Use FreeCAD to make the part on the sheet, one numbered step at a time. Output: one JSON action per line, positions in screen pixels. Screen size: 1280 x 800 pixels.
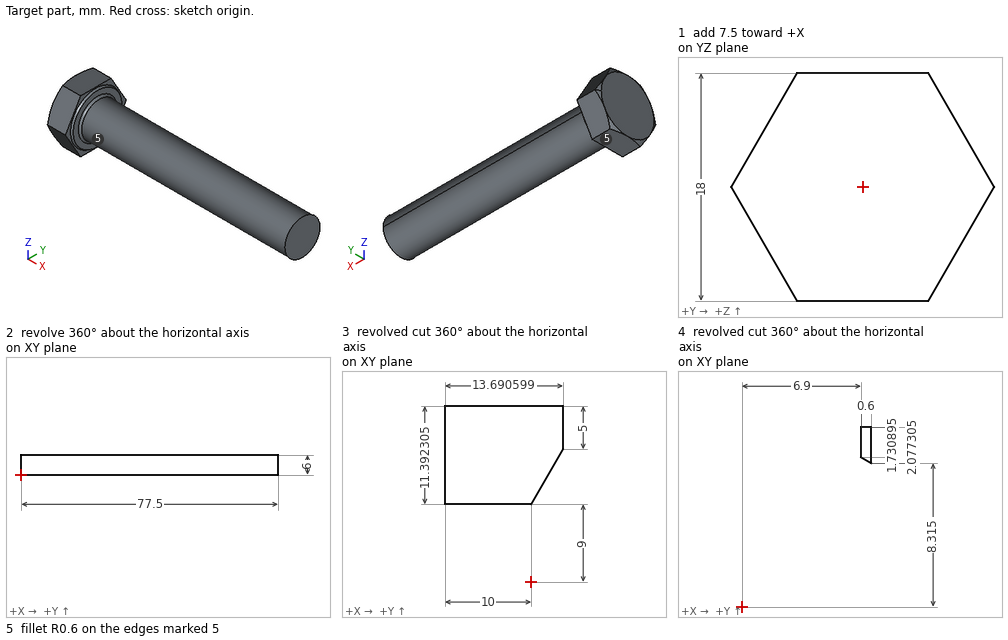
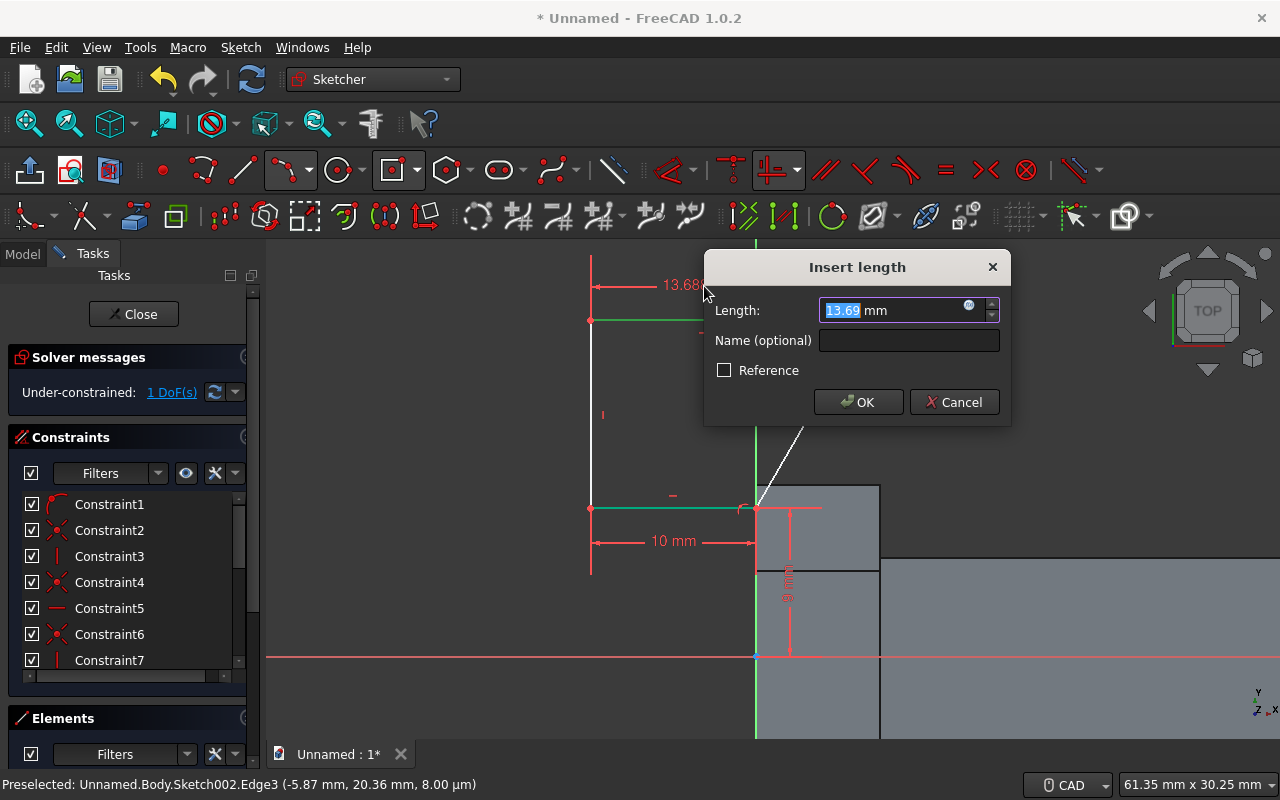
{"action": "type", "text": "13.690599"}
{"action": "key", "text": "Return"}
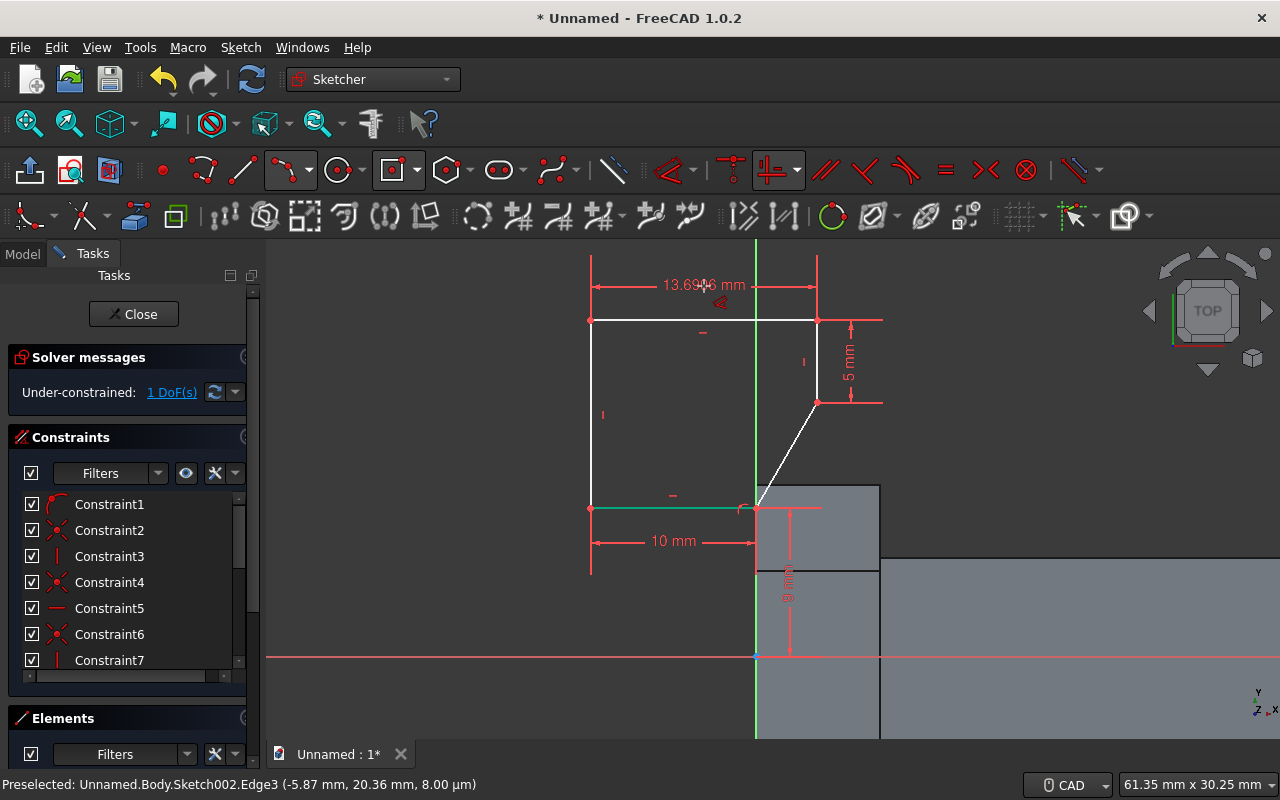
{"action": "left_click", "coordinate": [591, 377]}
{"action": "left_click", "coordinate": [557, 414]}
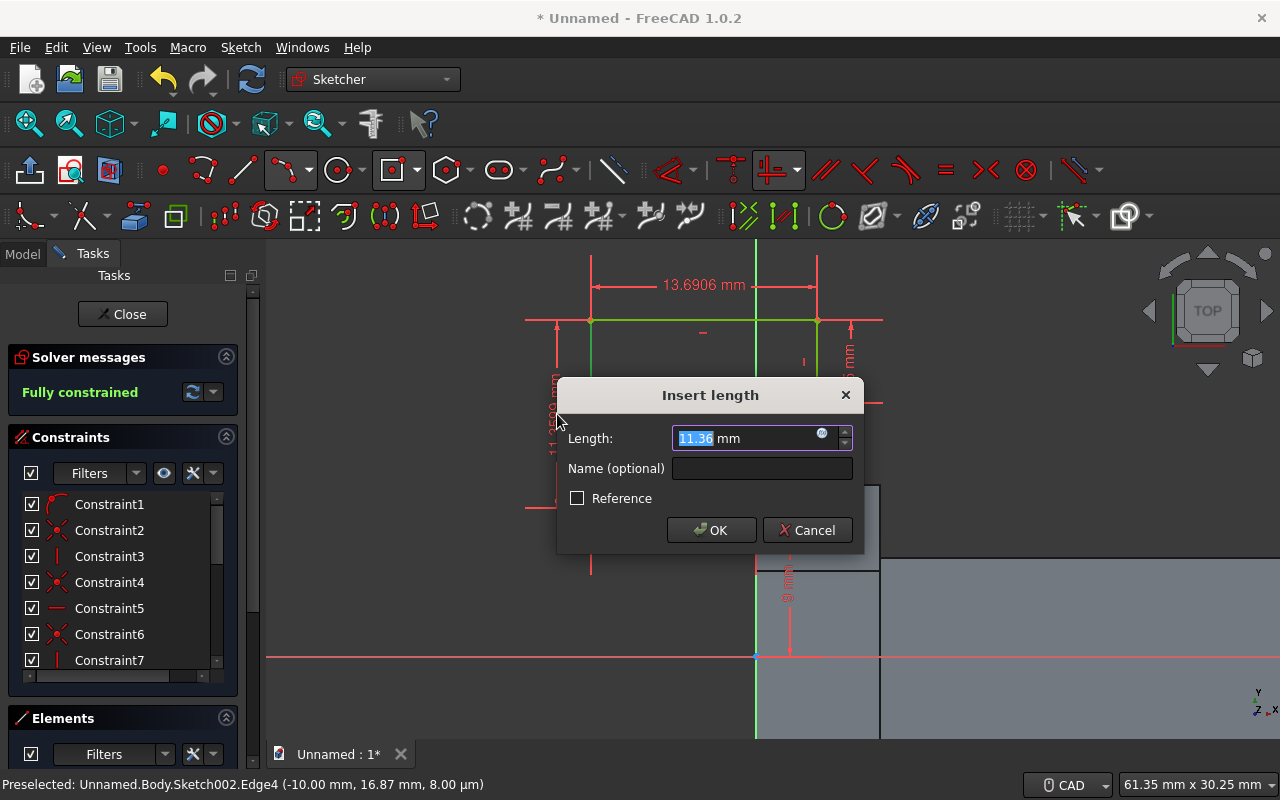
{"action": "type", "text": "11.392305"}
{"action": "key", "text": "Return"}
{"action": "key", "text": "Escape"}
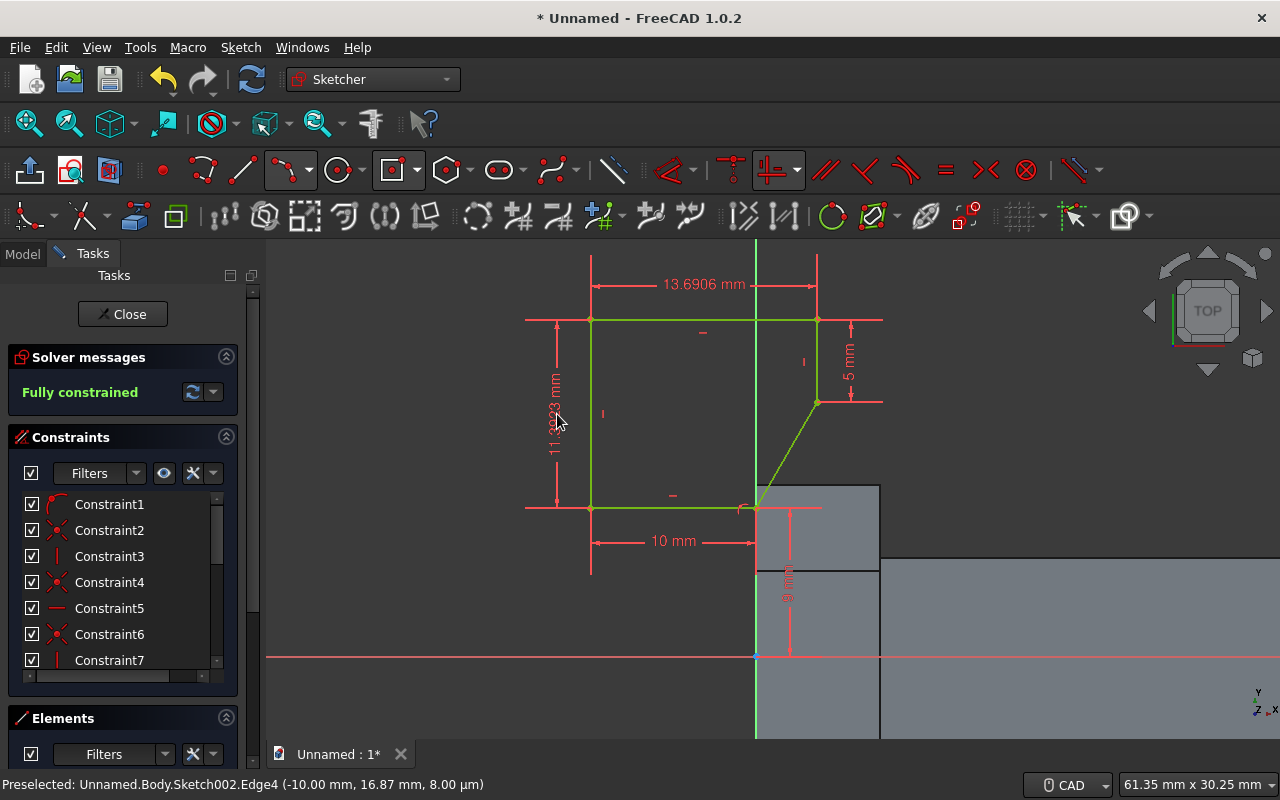
{"action": "left_click", "coordinate": [123, 314]}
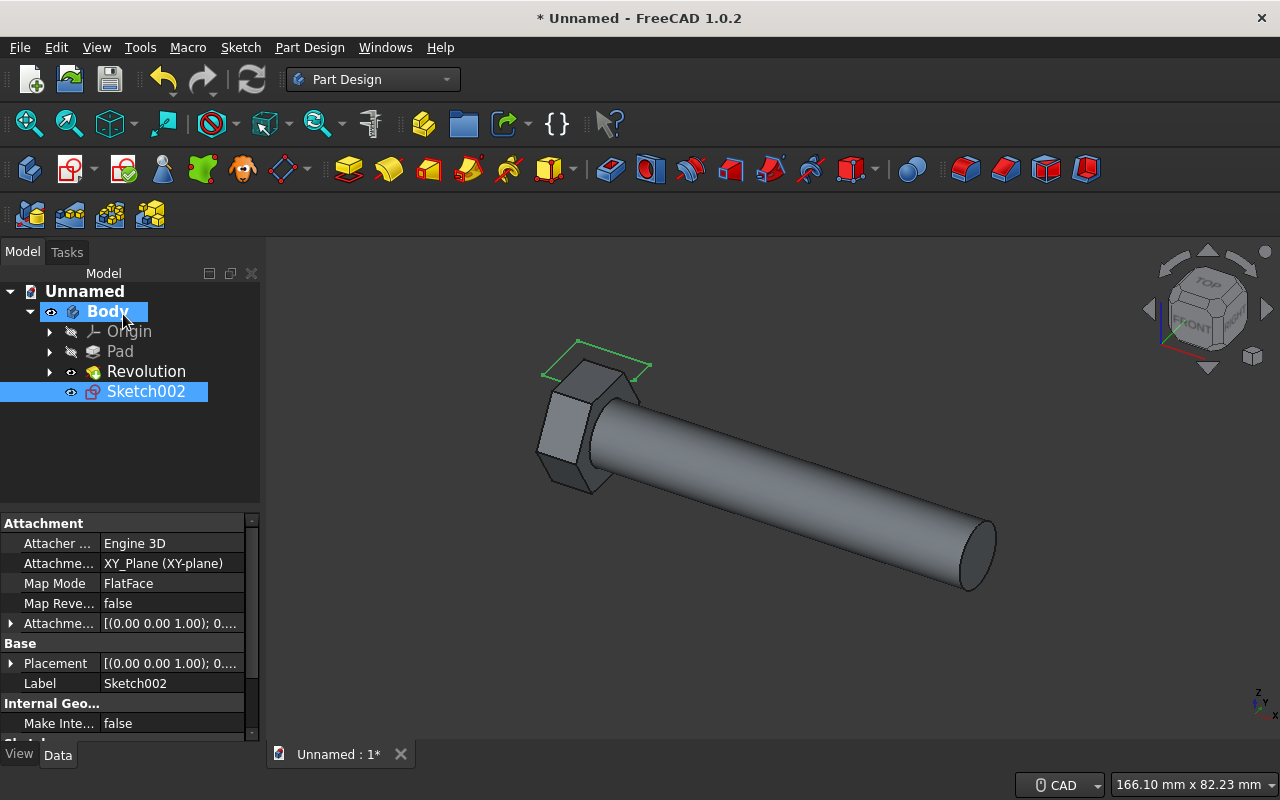
{"action": "left_click", "coordinate": [692, 170]}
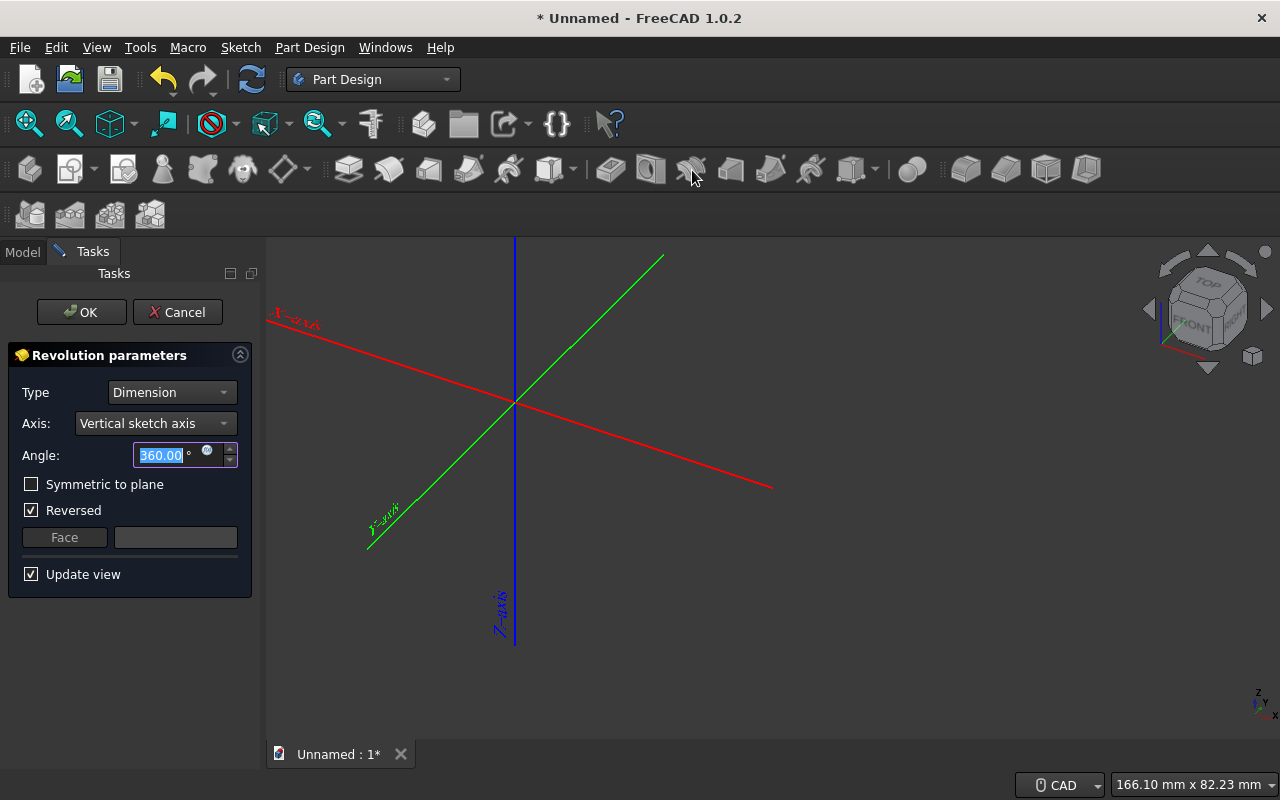
{"action": "left_click", "coordinate": [156, 424]}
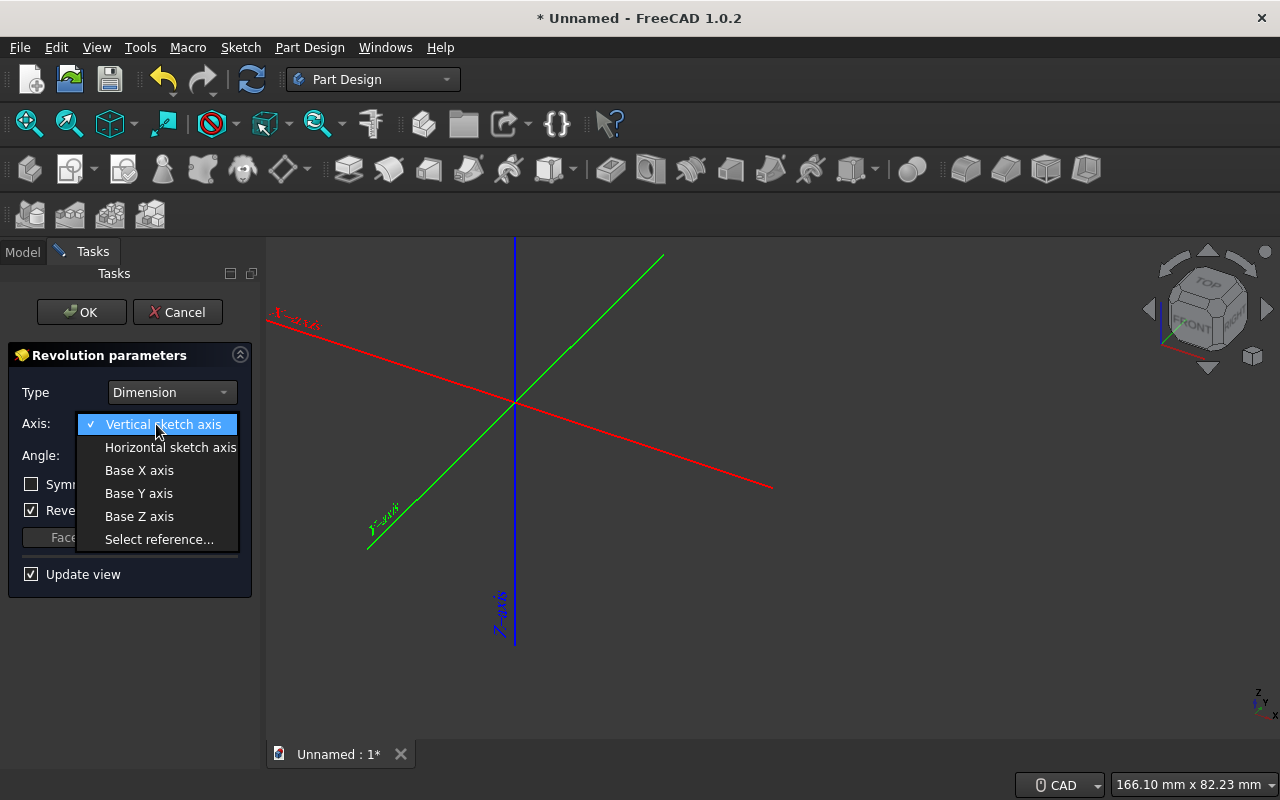
{"action": "left_click", "coordinate": [156, 448]}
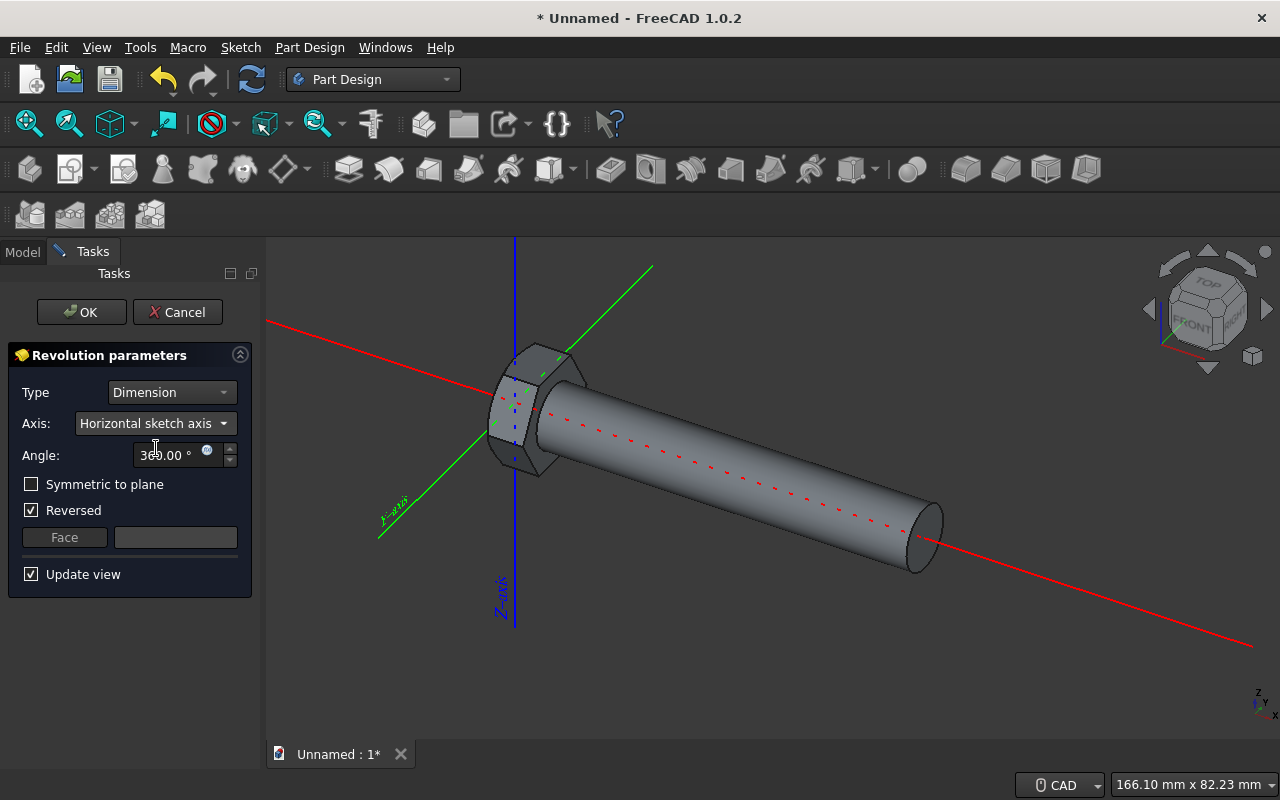
{"action": "left_click", "coordinate": [82, 312]}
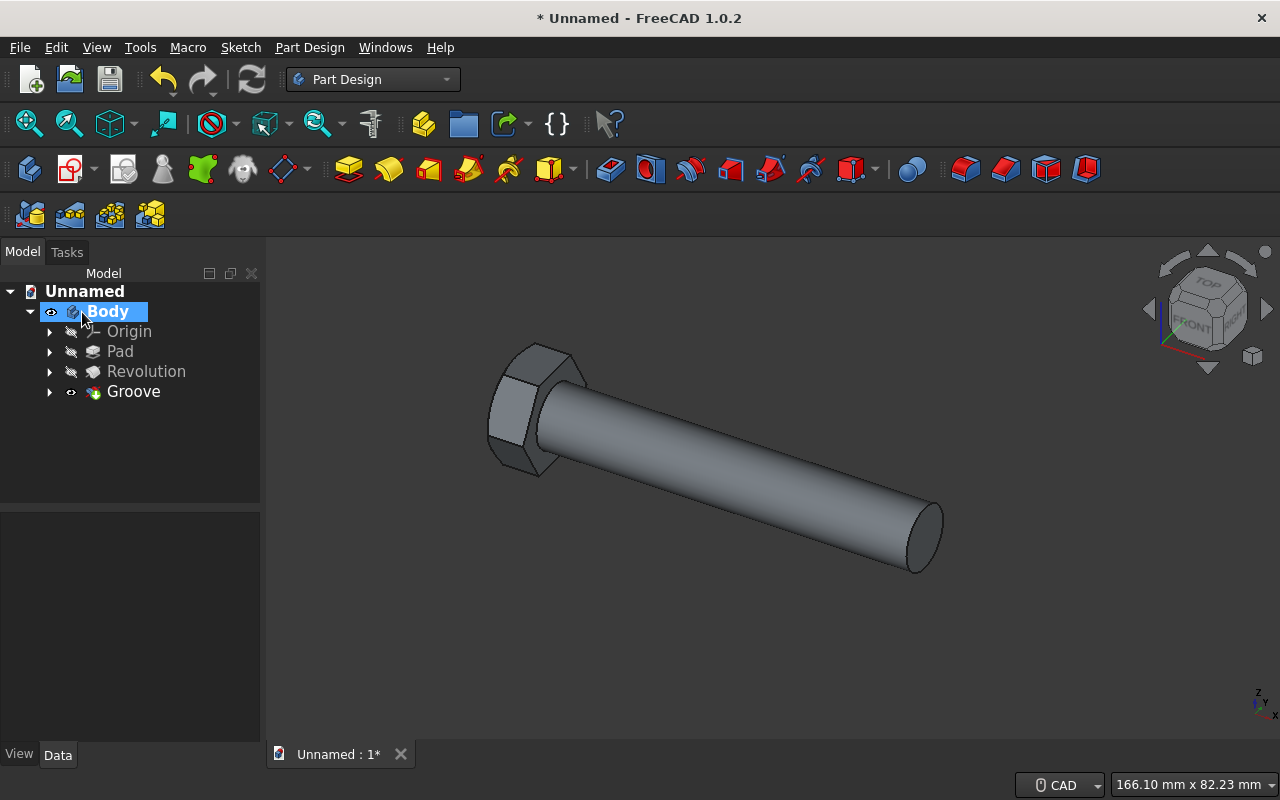
{"action": "left_click", "coordinate": [70, 170]}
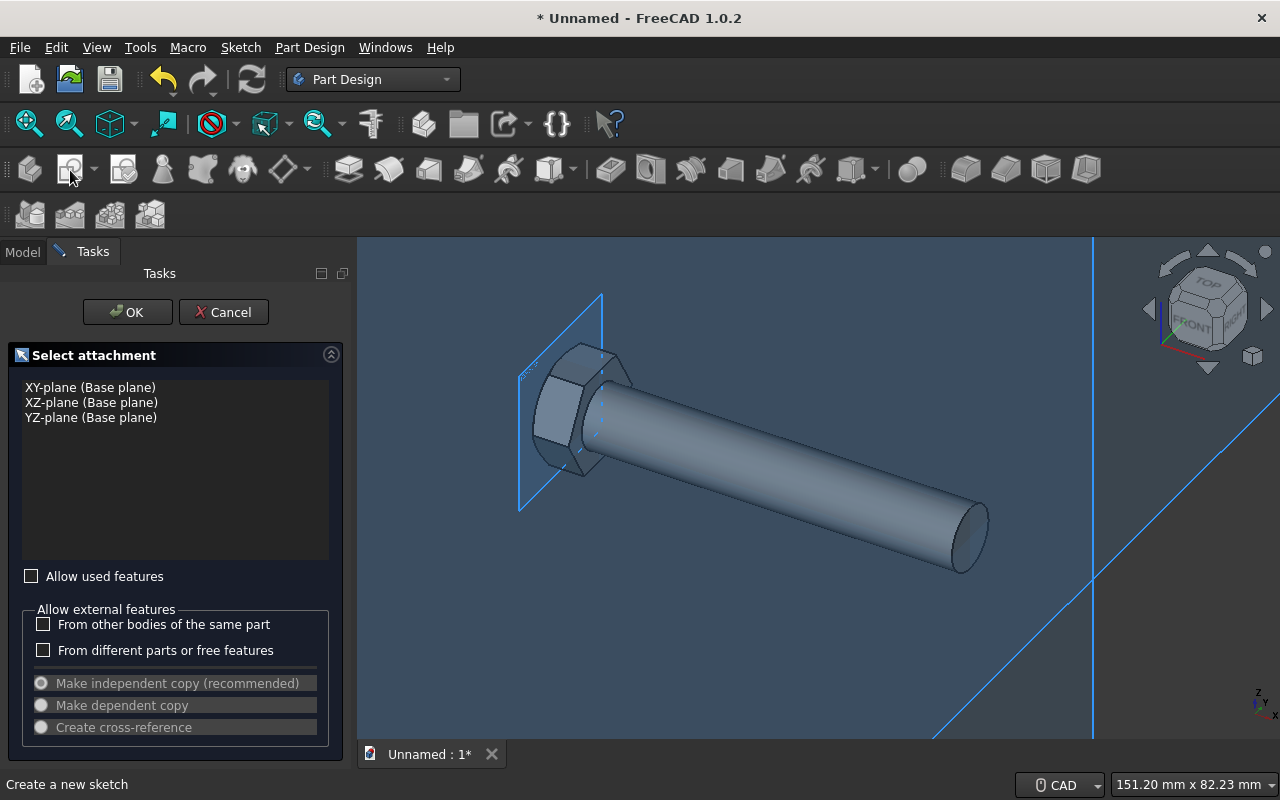
{"action": "left_click", "coordinate": [82, 388]}